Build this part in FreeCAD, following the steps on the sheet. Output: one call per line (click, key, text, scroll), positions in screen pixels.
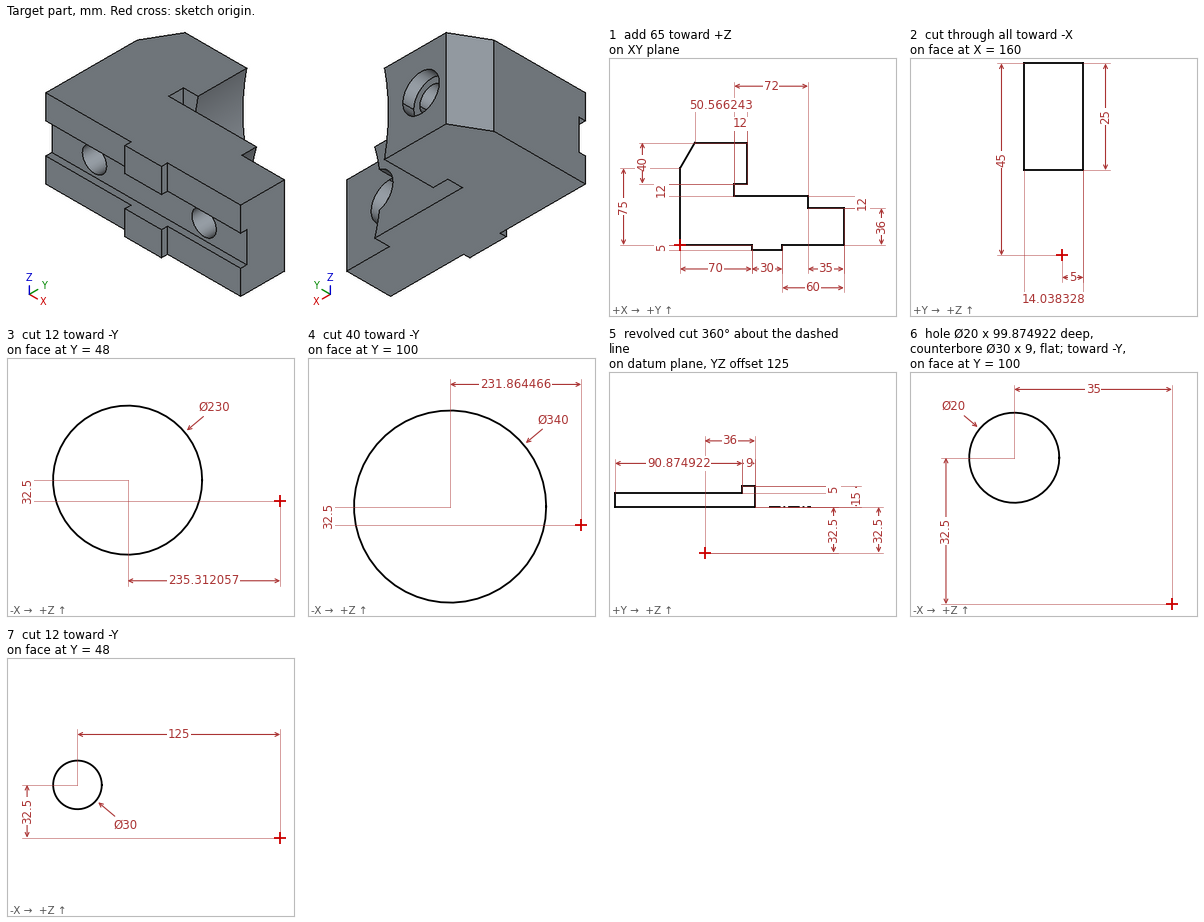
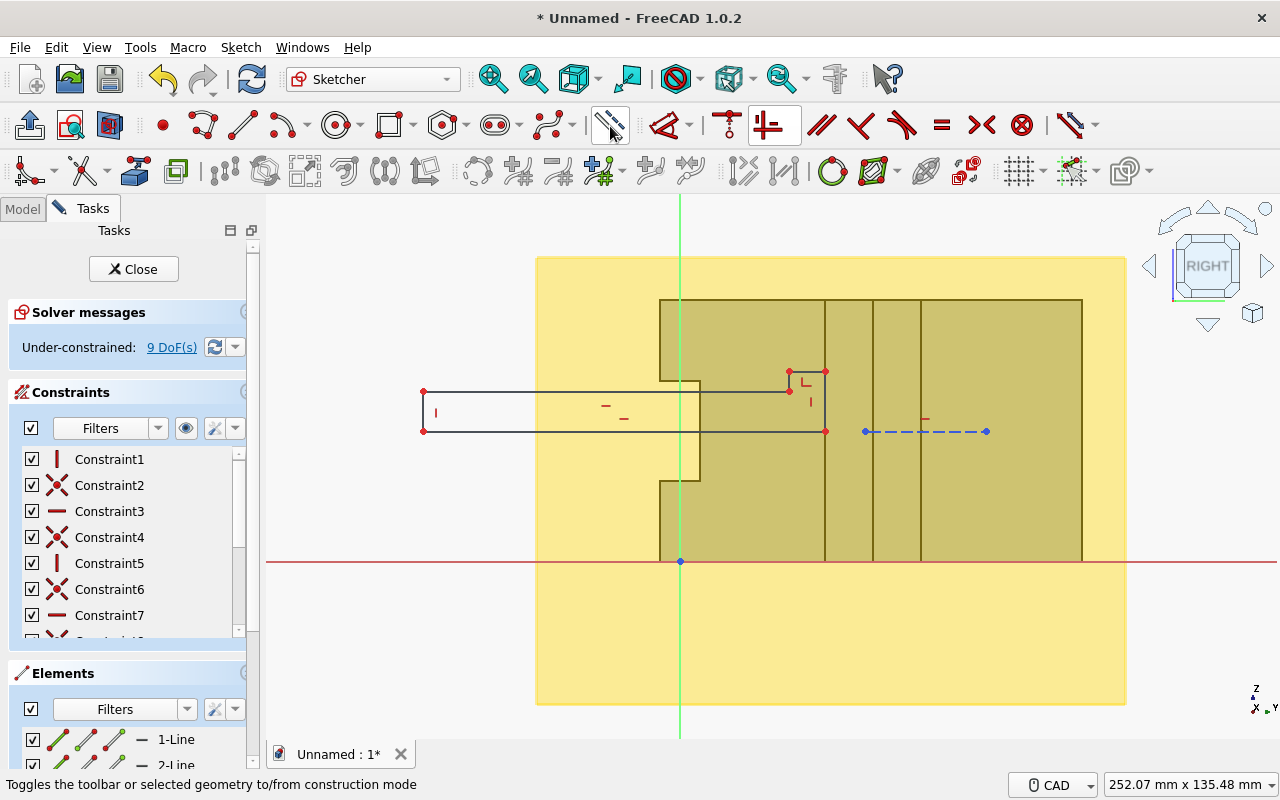
click(664, 126)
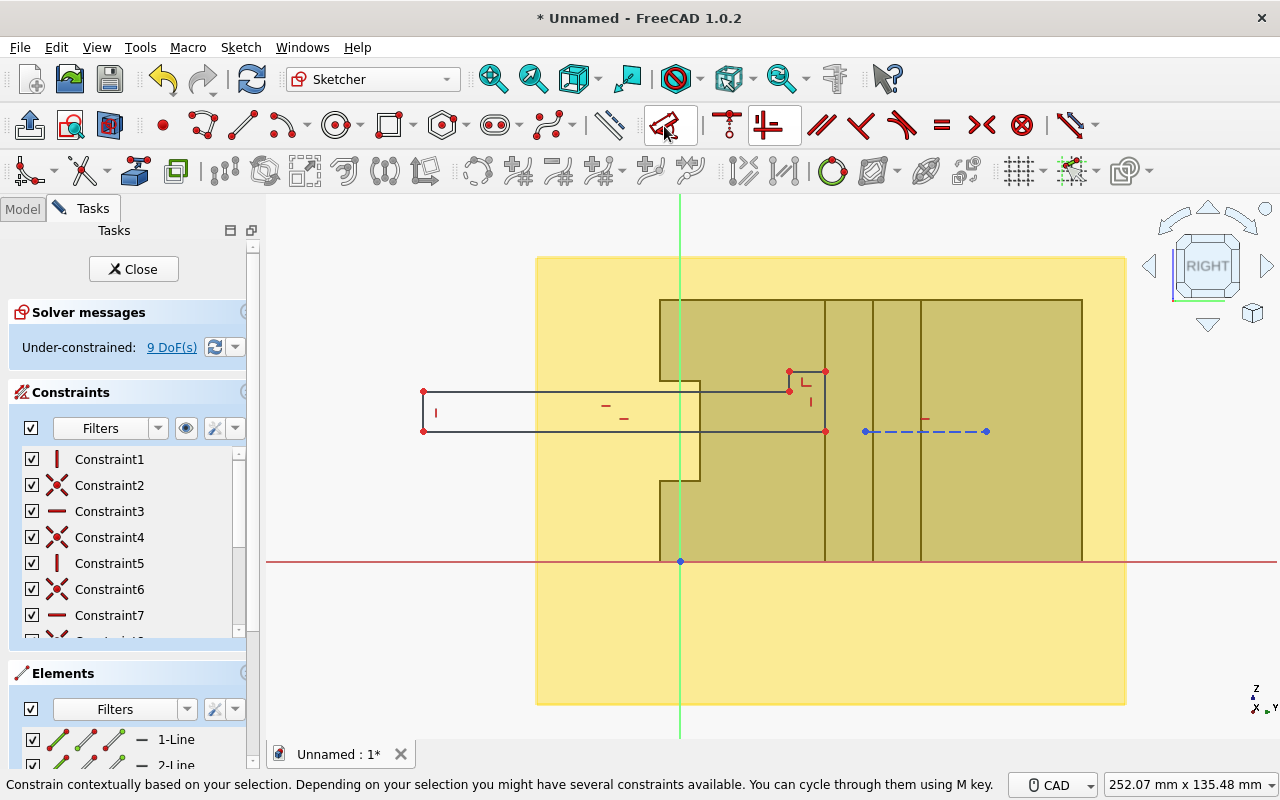
scroll(814, 372, up, 2)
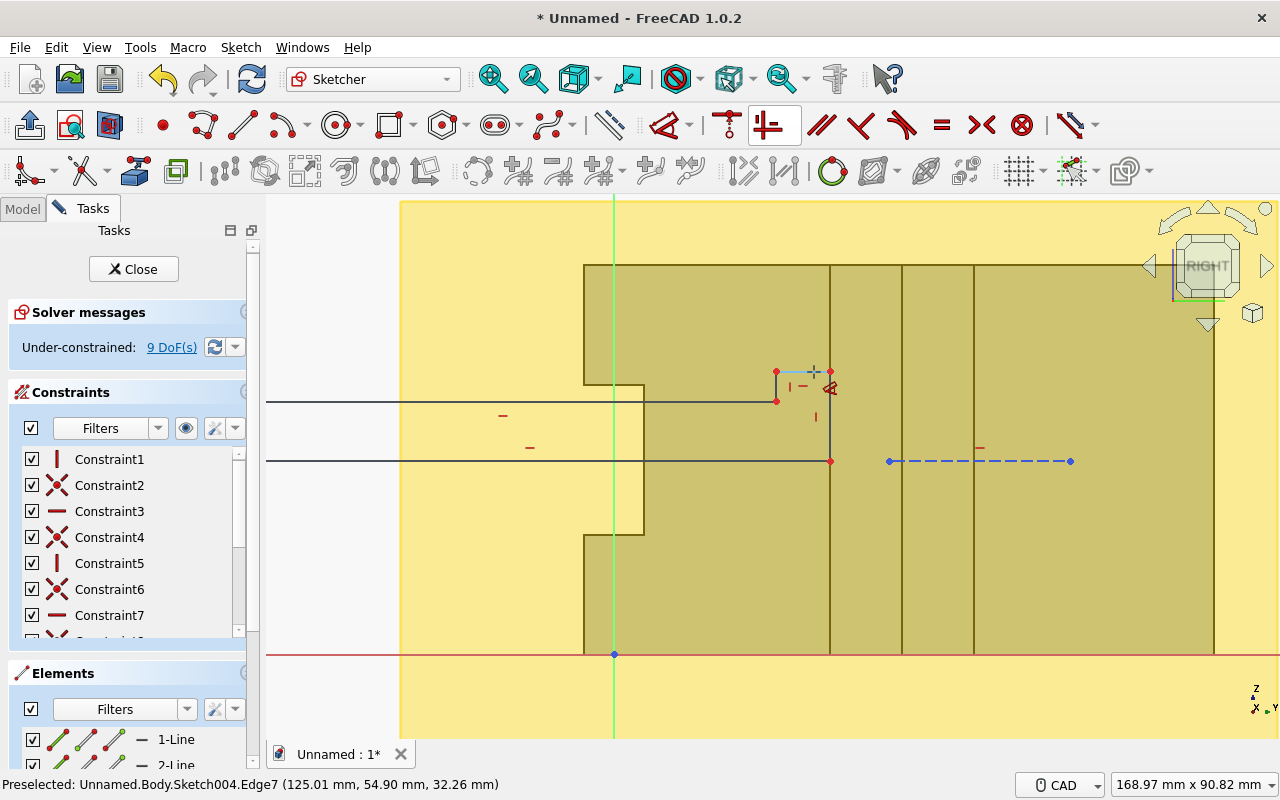
click(814, 372)
click(803, 338)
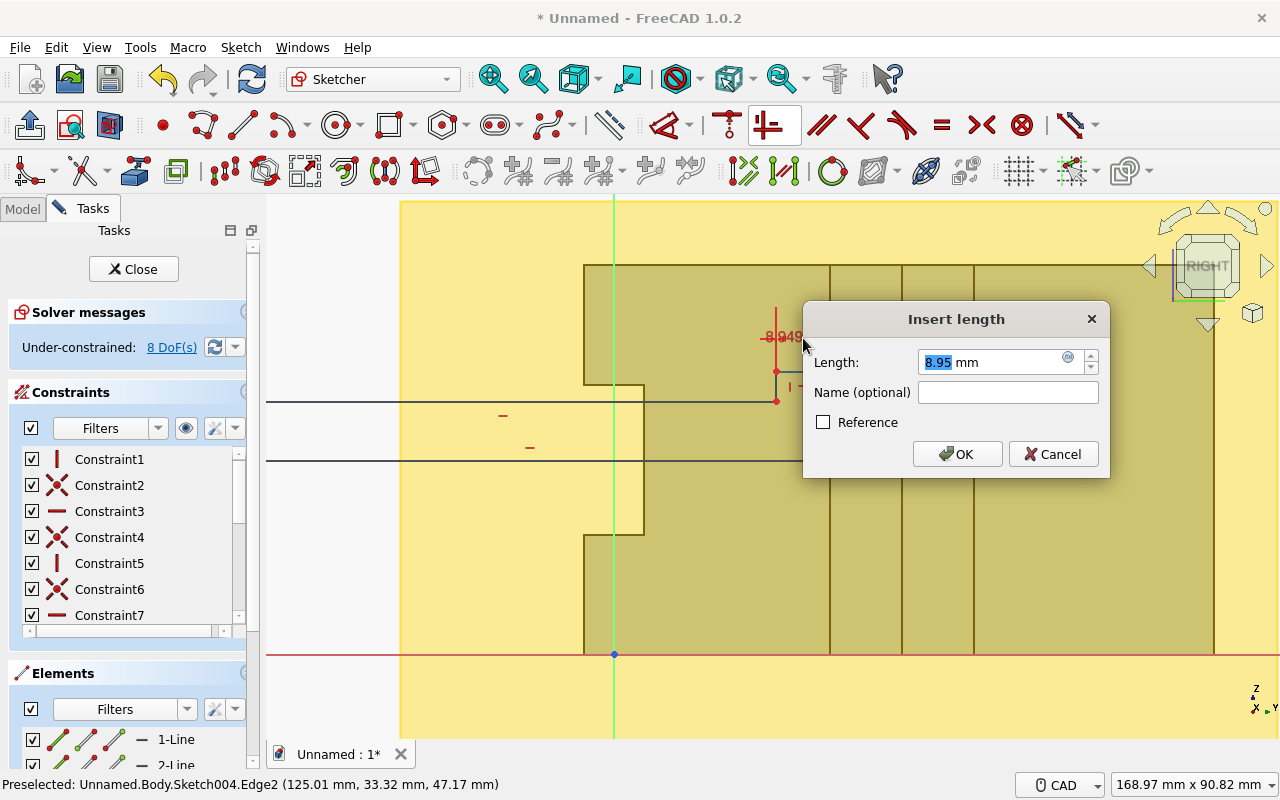
text(9)
key(Return)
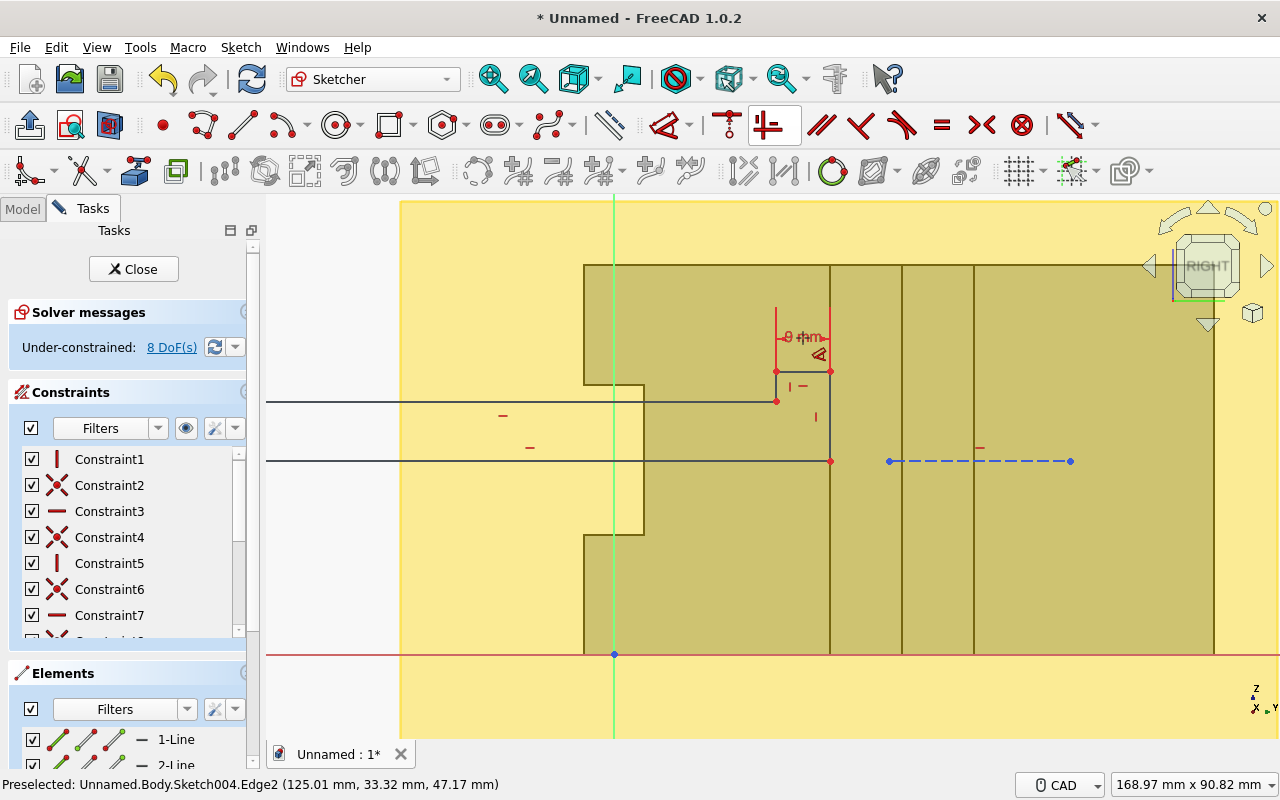
scroll(776, 384, up, 2)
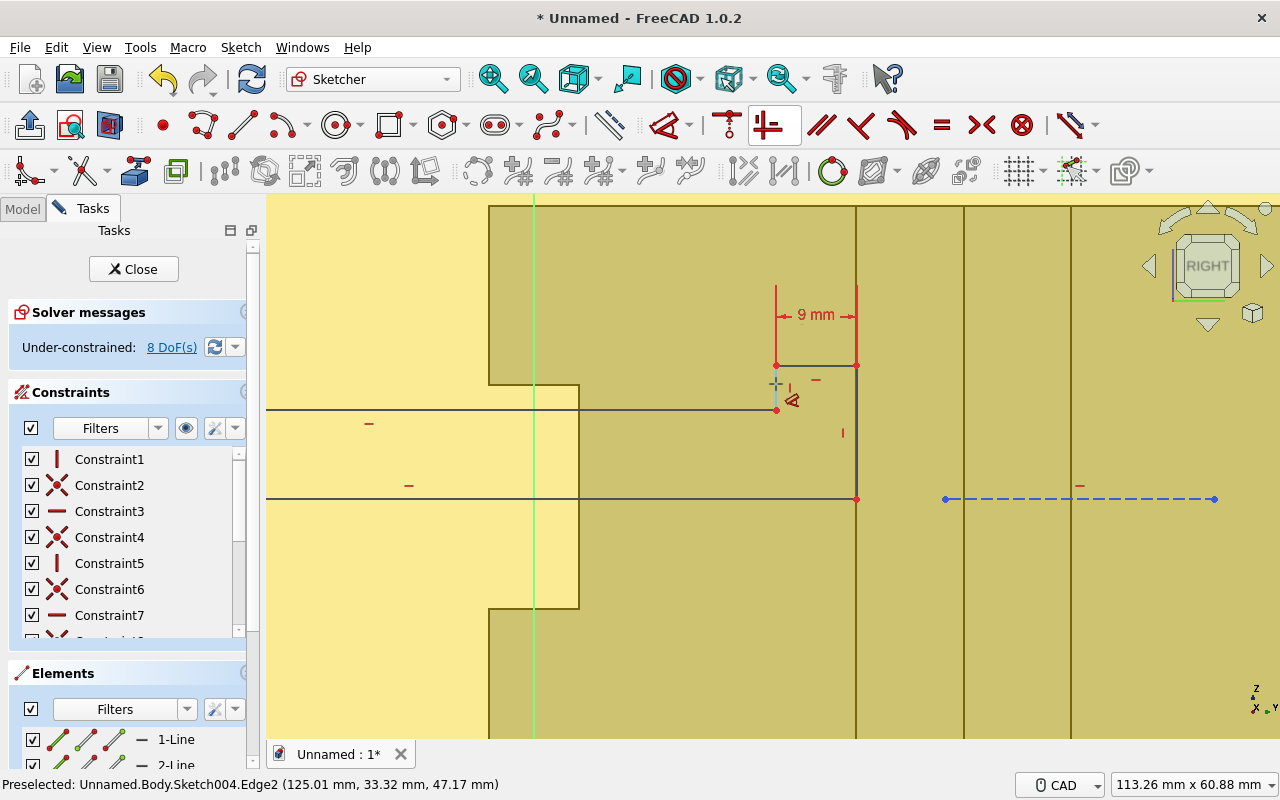
click(776, 383)
click(810, 388)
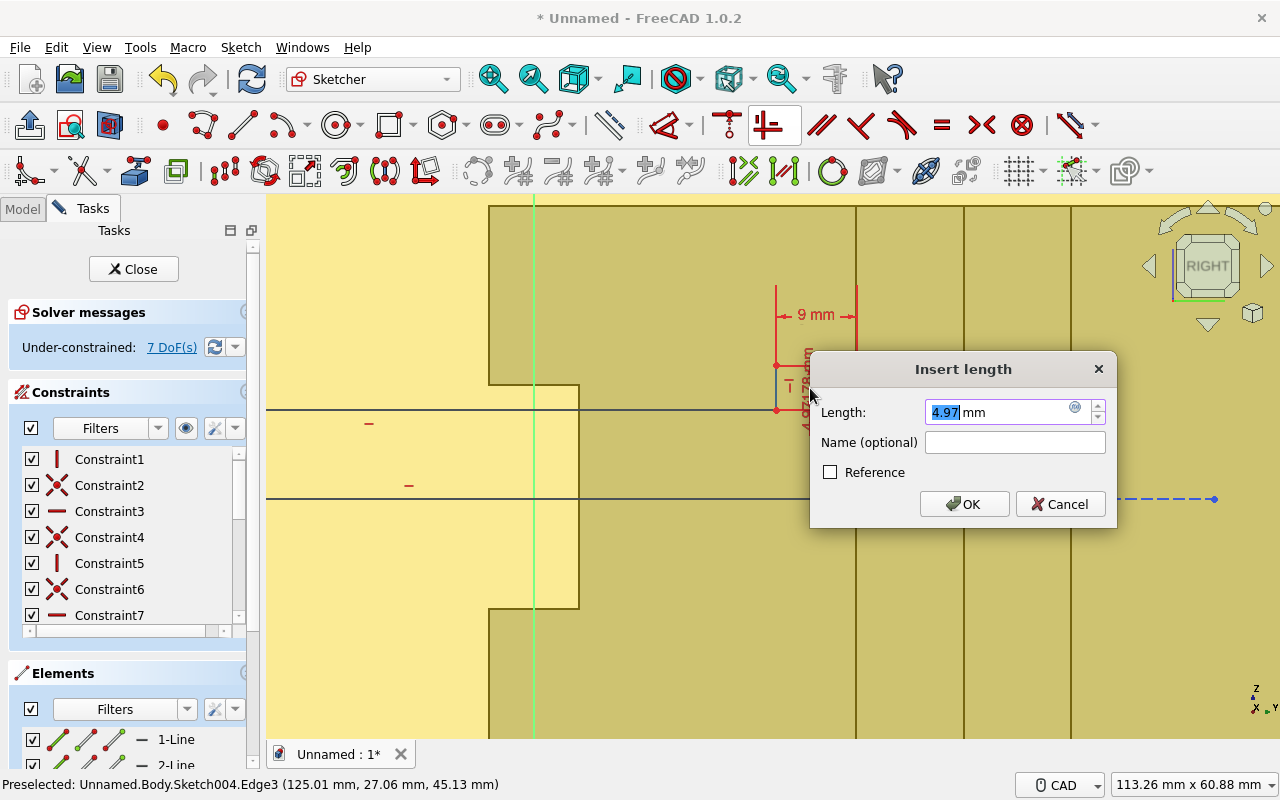
text(5)
key(Return)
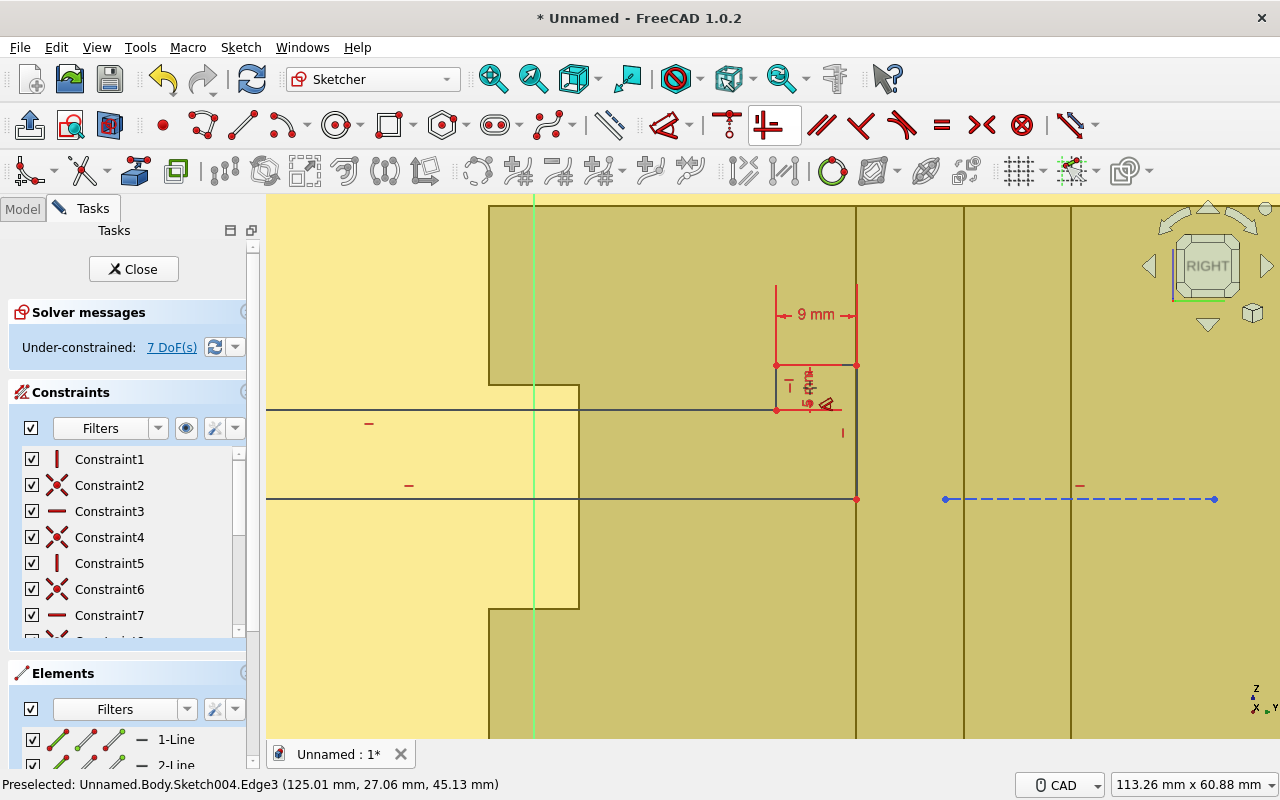
click(857, 459)
click(891, 432)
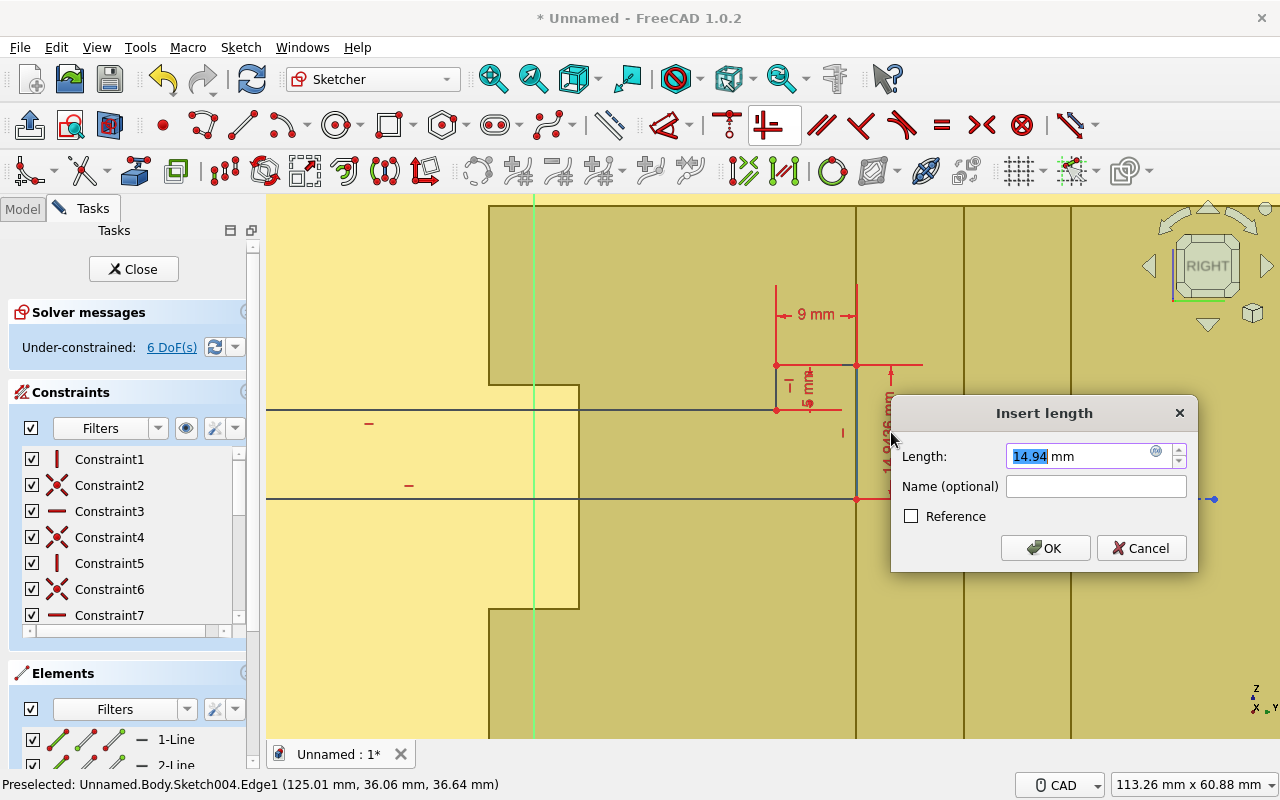
text(15)
key(Return)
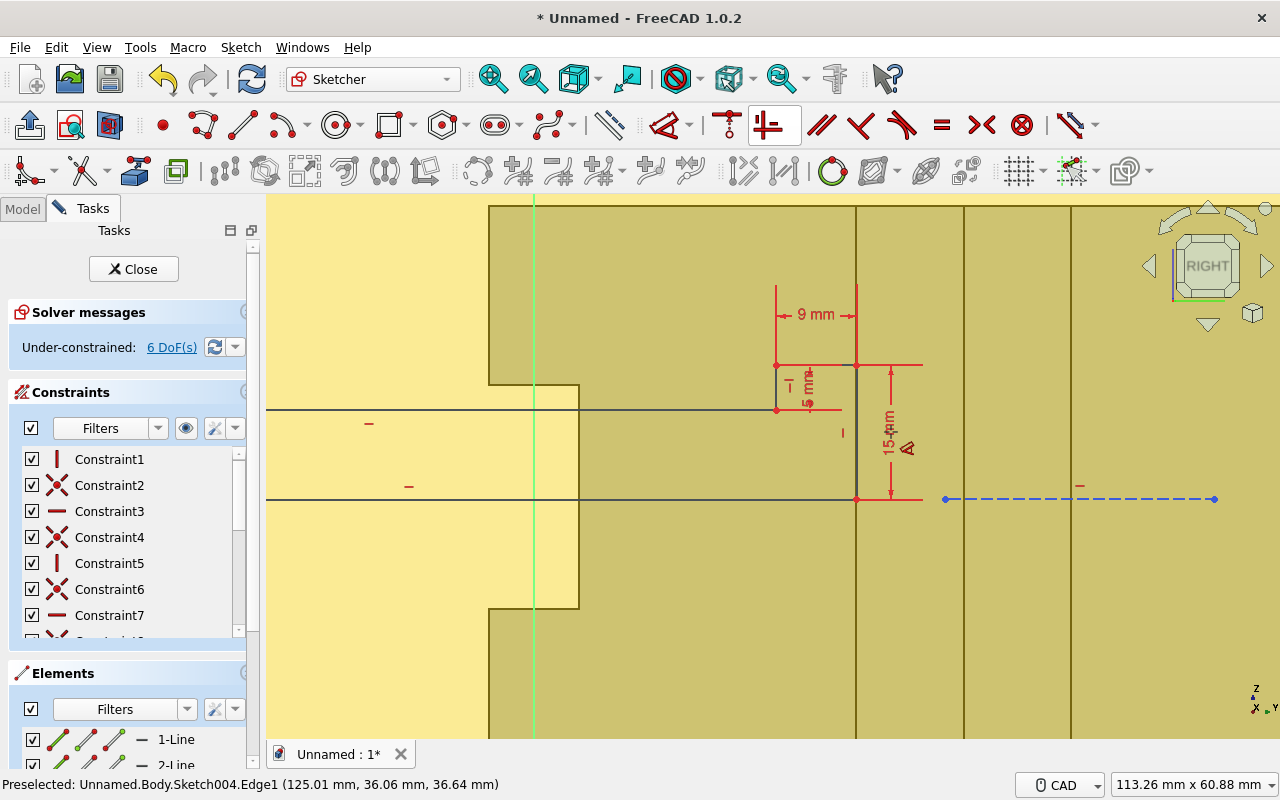
click(857, 500)
click(696, 466)